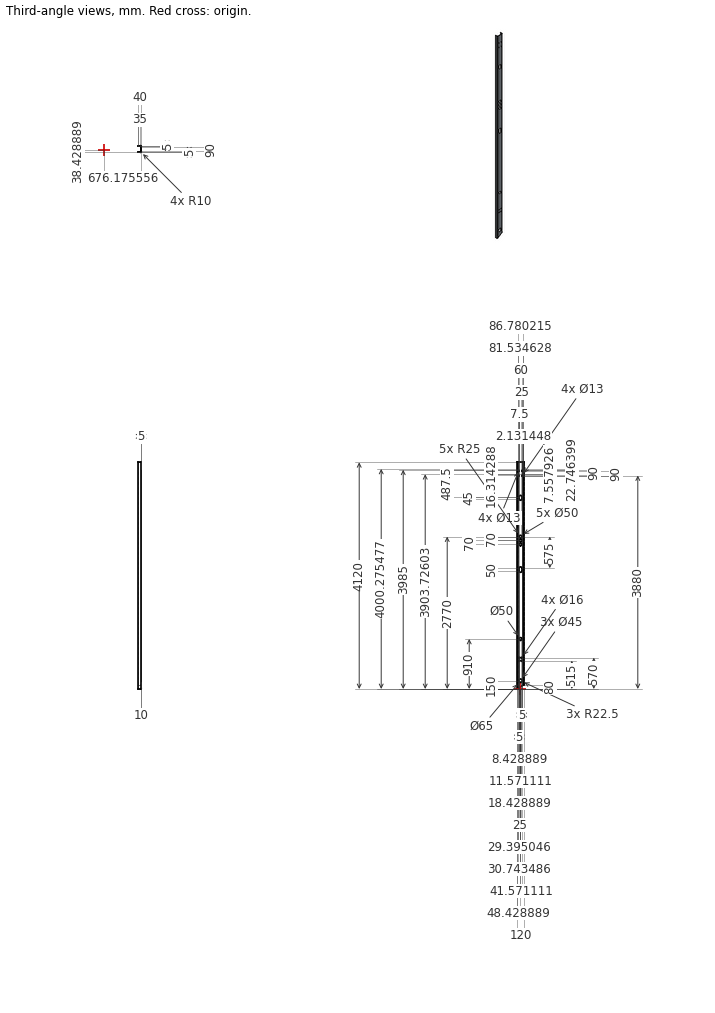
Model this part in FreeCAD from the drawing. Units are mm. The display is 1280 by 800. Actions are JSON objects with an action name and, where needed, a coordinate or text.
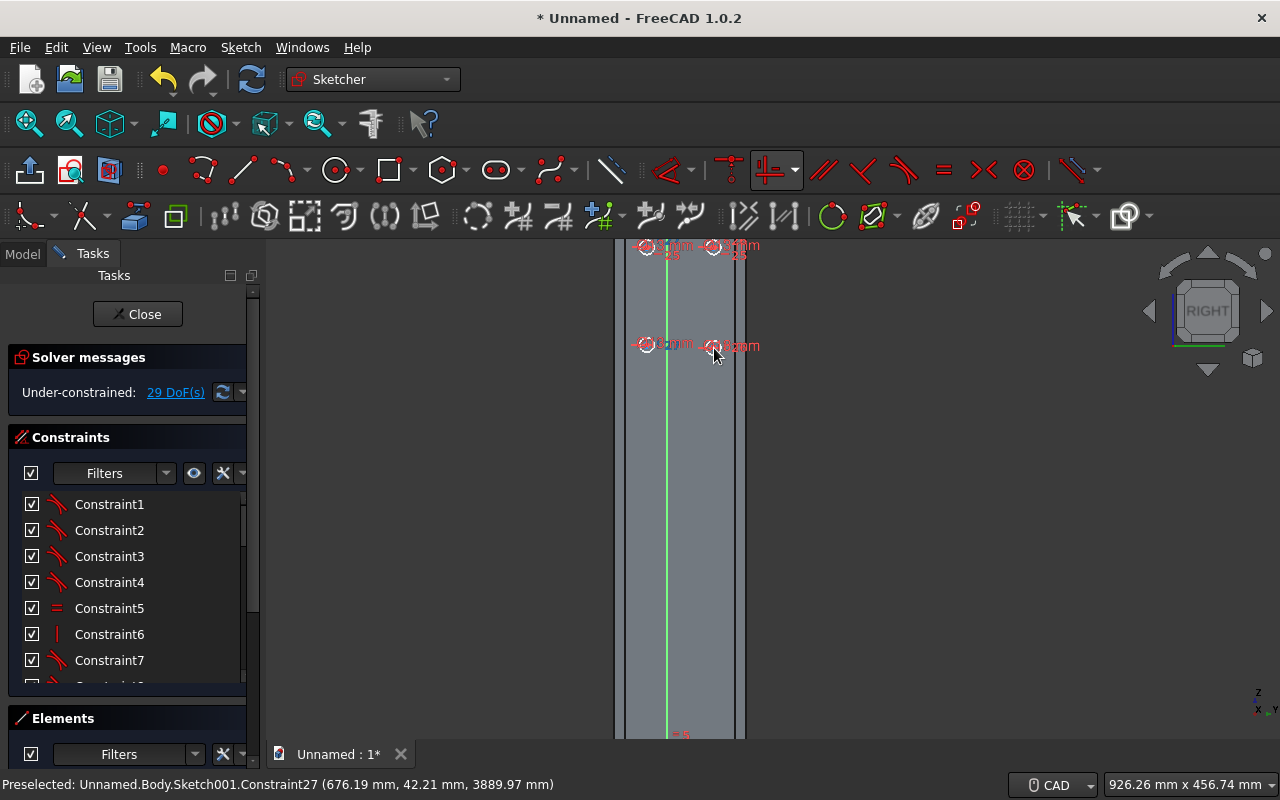
{"action": "left_click", "coordinate": [714, 348]}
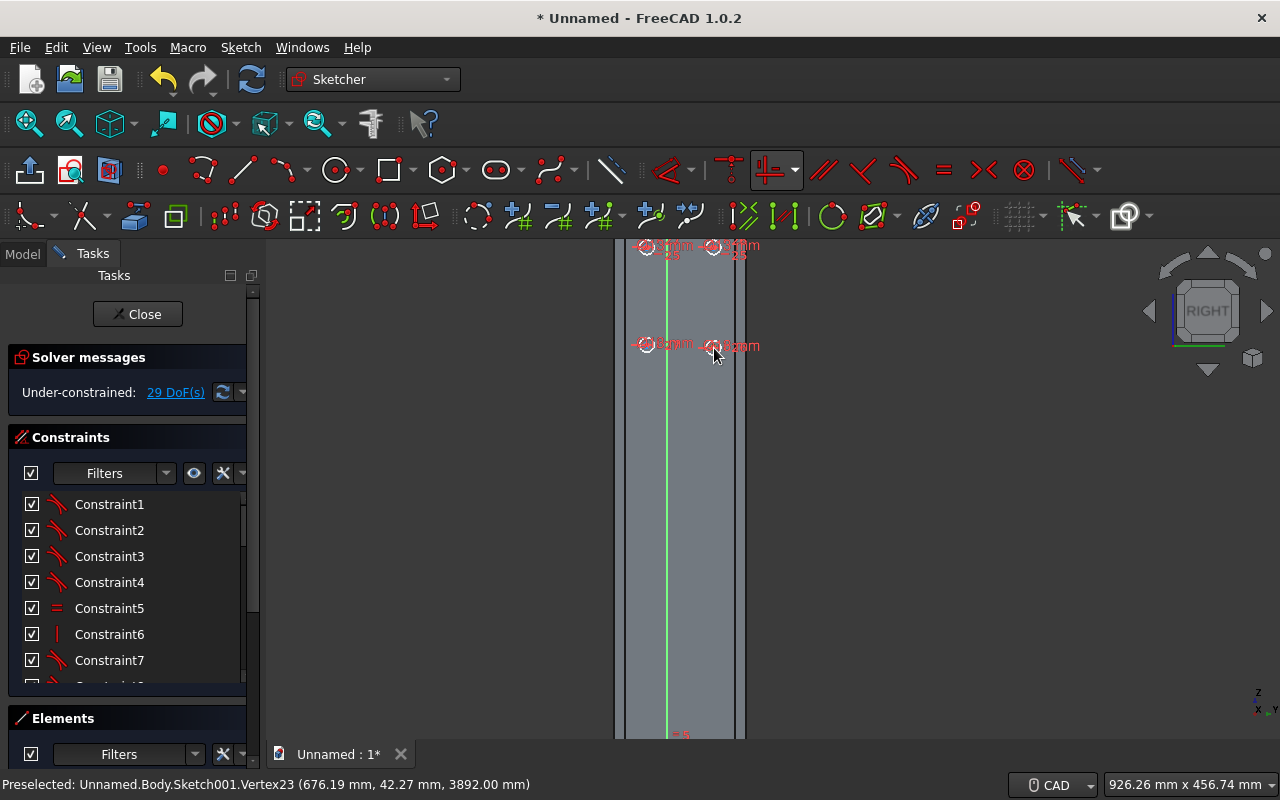
{"action": "scroll", "coordinate": [706, 334], "scroll_direction": "down", "scroll_amount": 13}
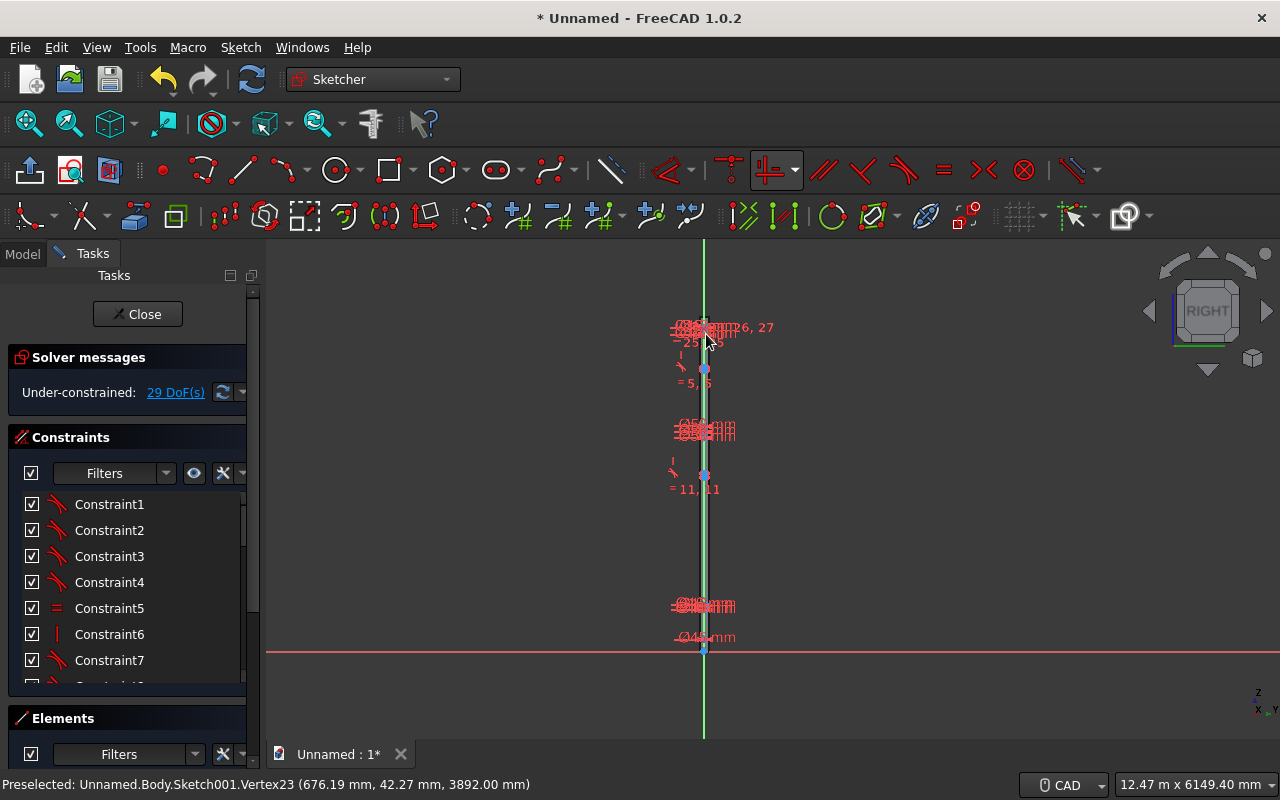
{"action": "scroll", "coordinate": [702, 335], "scroll_direction": "up", "scroll_amount": 5}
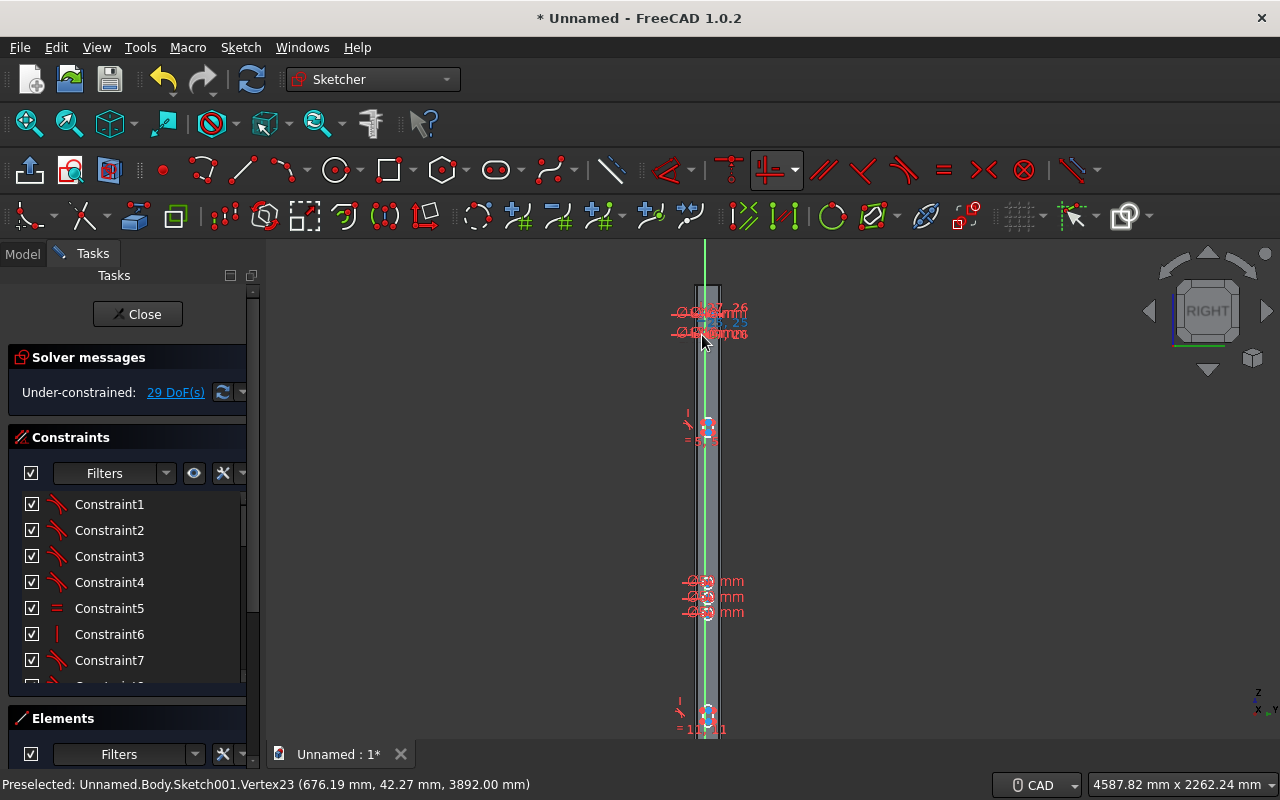
{"action": "scroll", "coordinate": [701, 335], "scroll_direction": "up", "scroll_amount": 4}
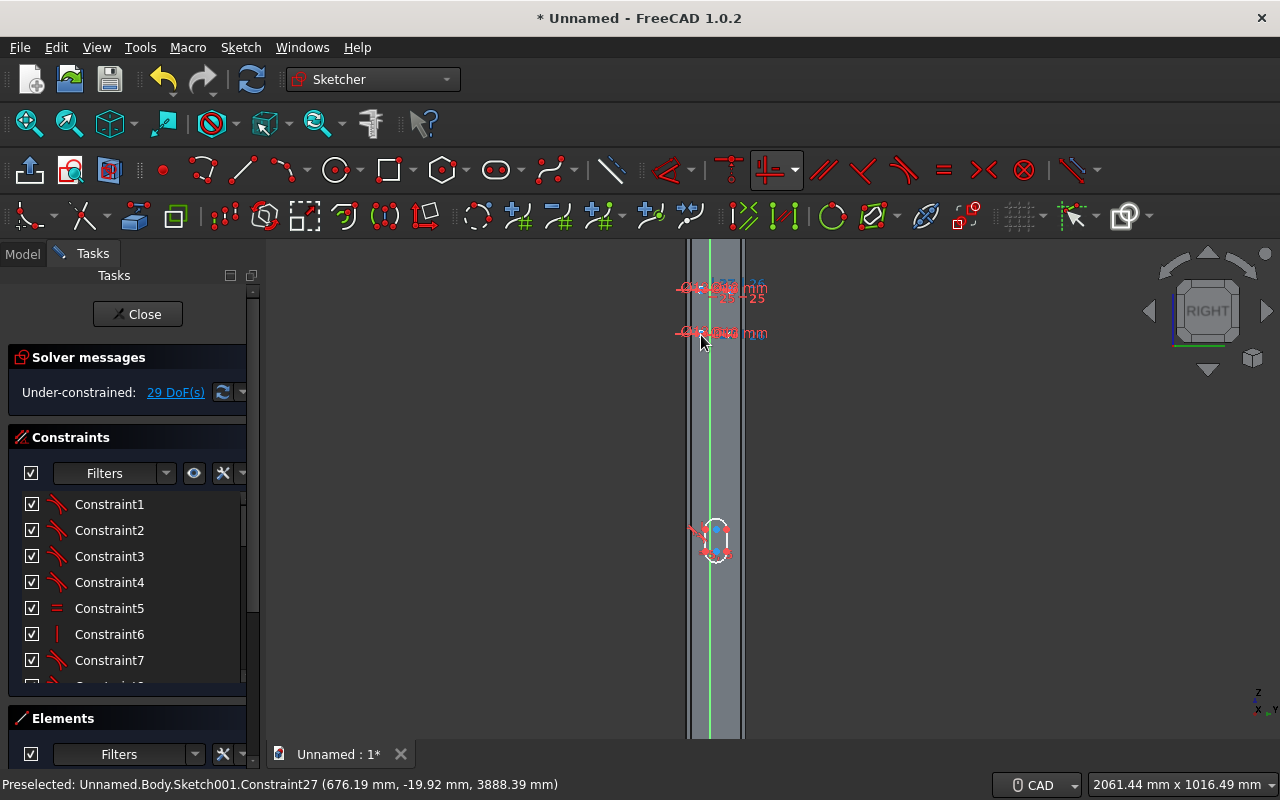
{"action": "left_click", "coordinate": [701, 334]}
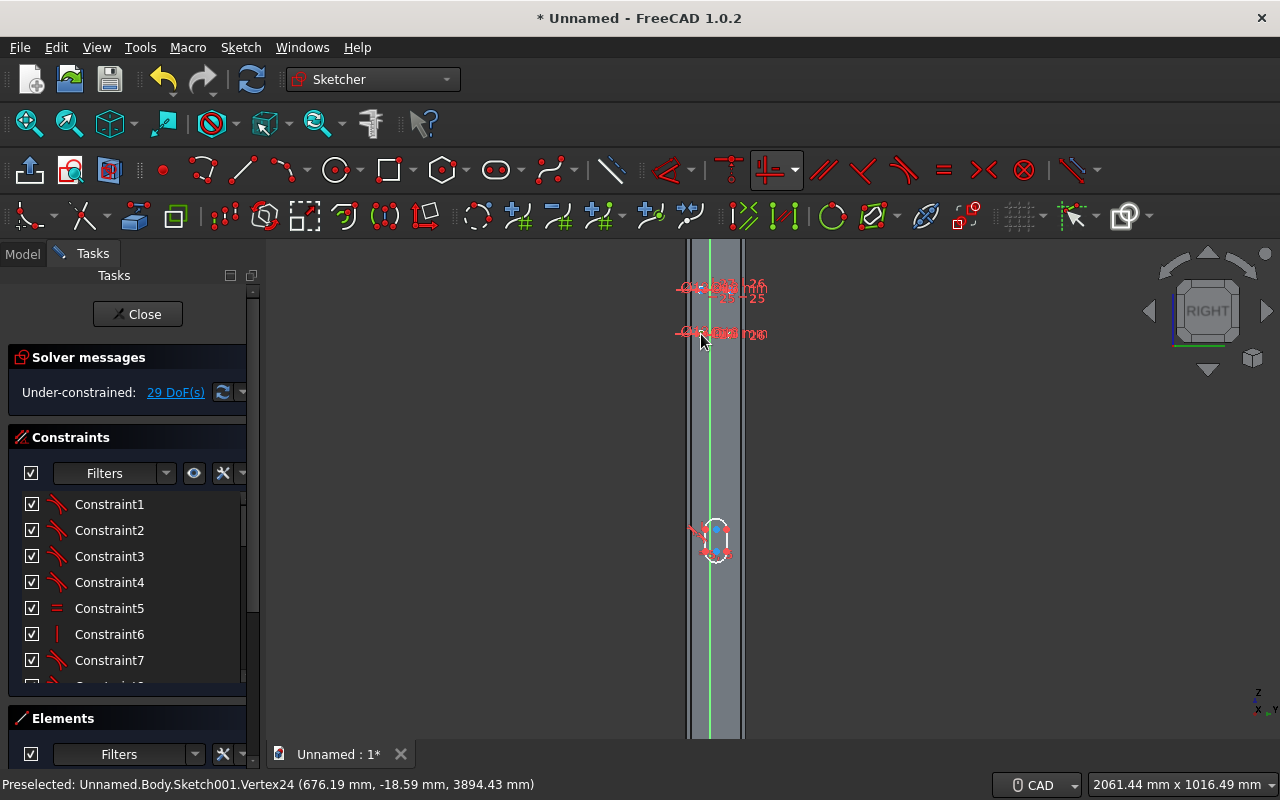
{"action": "left_click", "coordinate": [798, 170]}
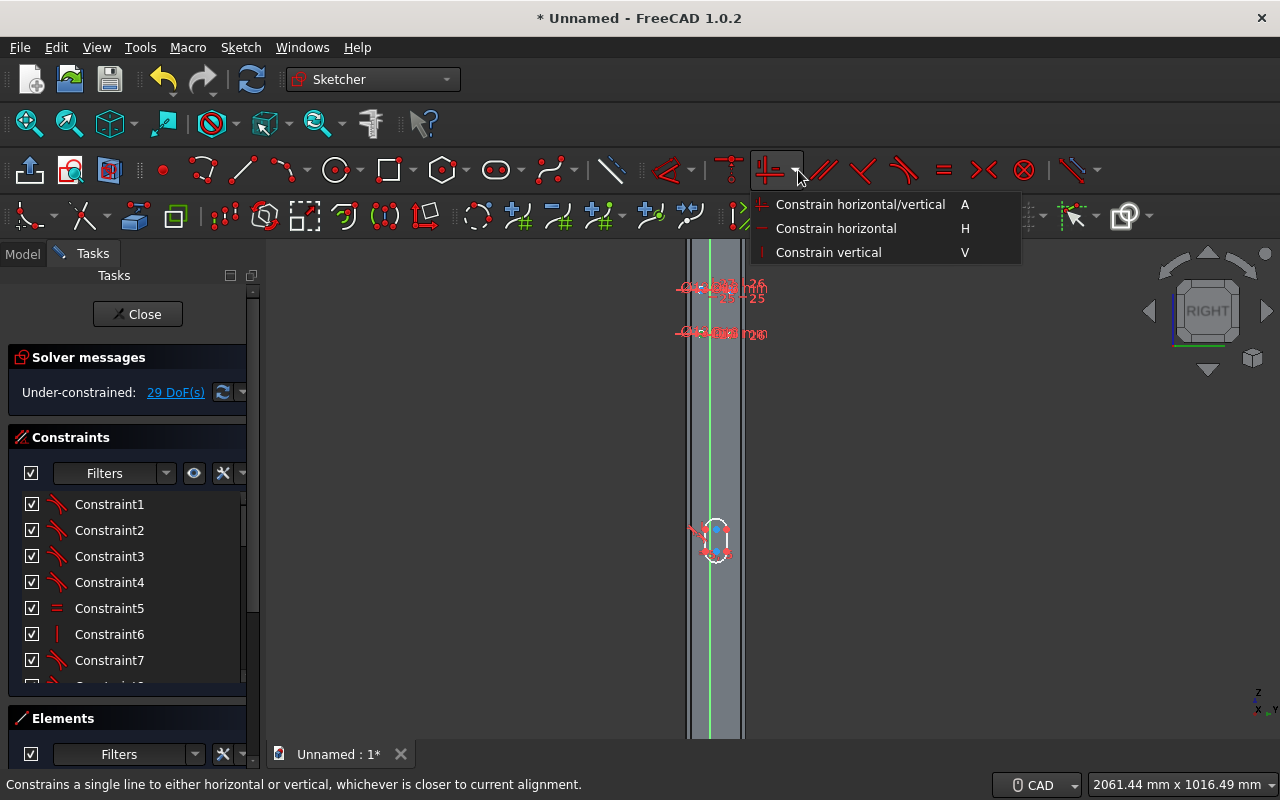
{"action": "left_click", "coordinate": [886, 228]}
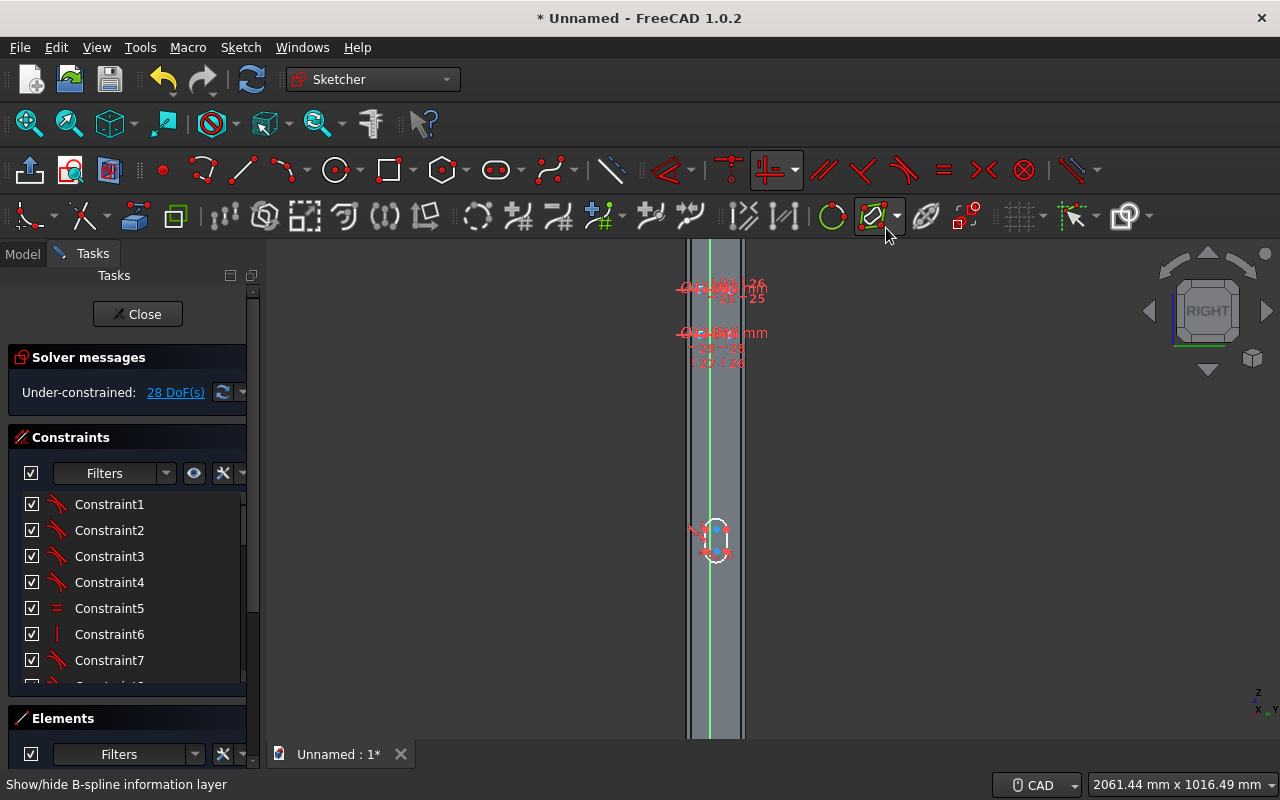
{"action": "scroll", "coordinate": [702, 335], "scroll_direction": "down", "scroll_amount": 9}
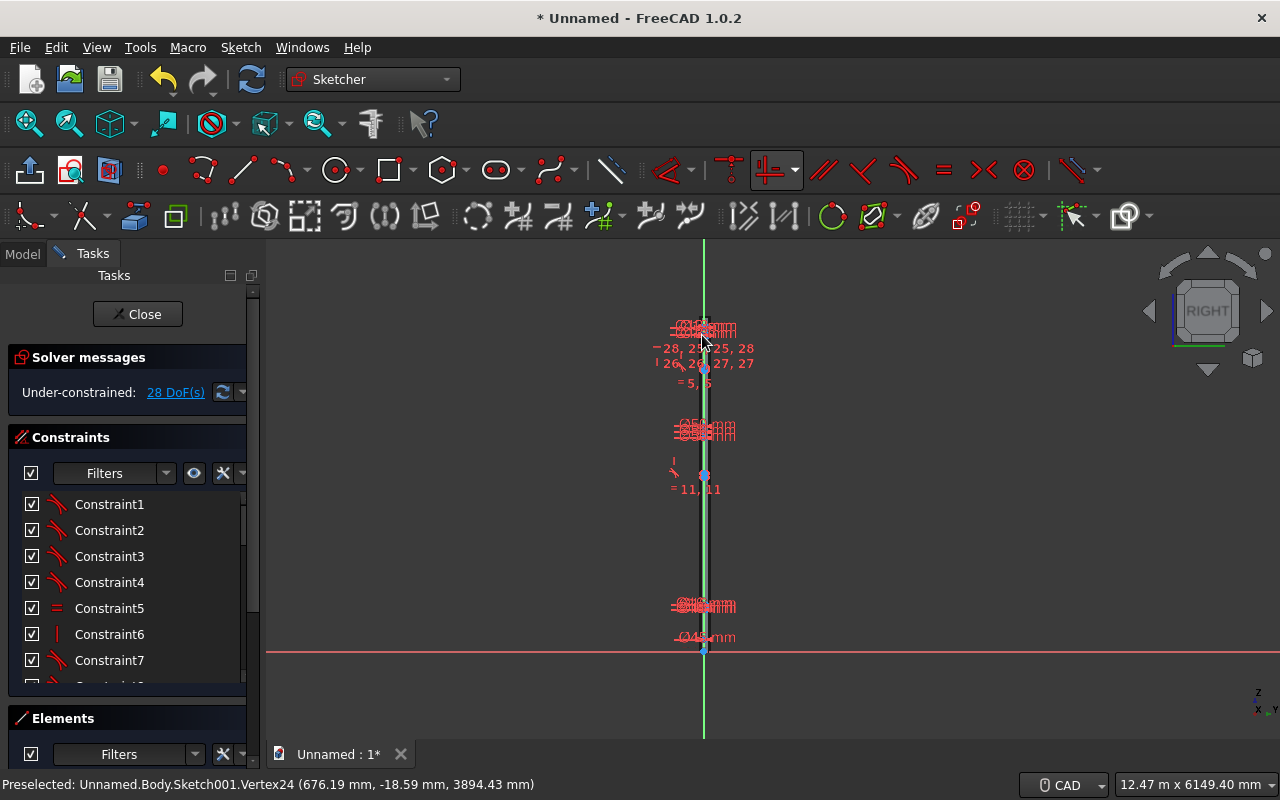
{"action": "scroll", "coordinate": [705, 426], "scroll_direction": "up", "scroll_amount": 4}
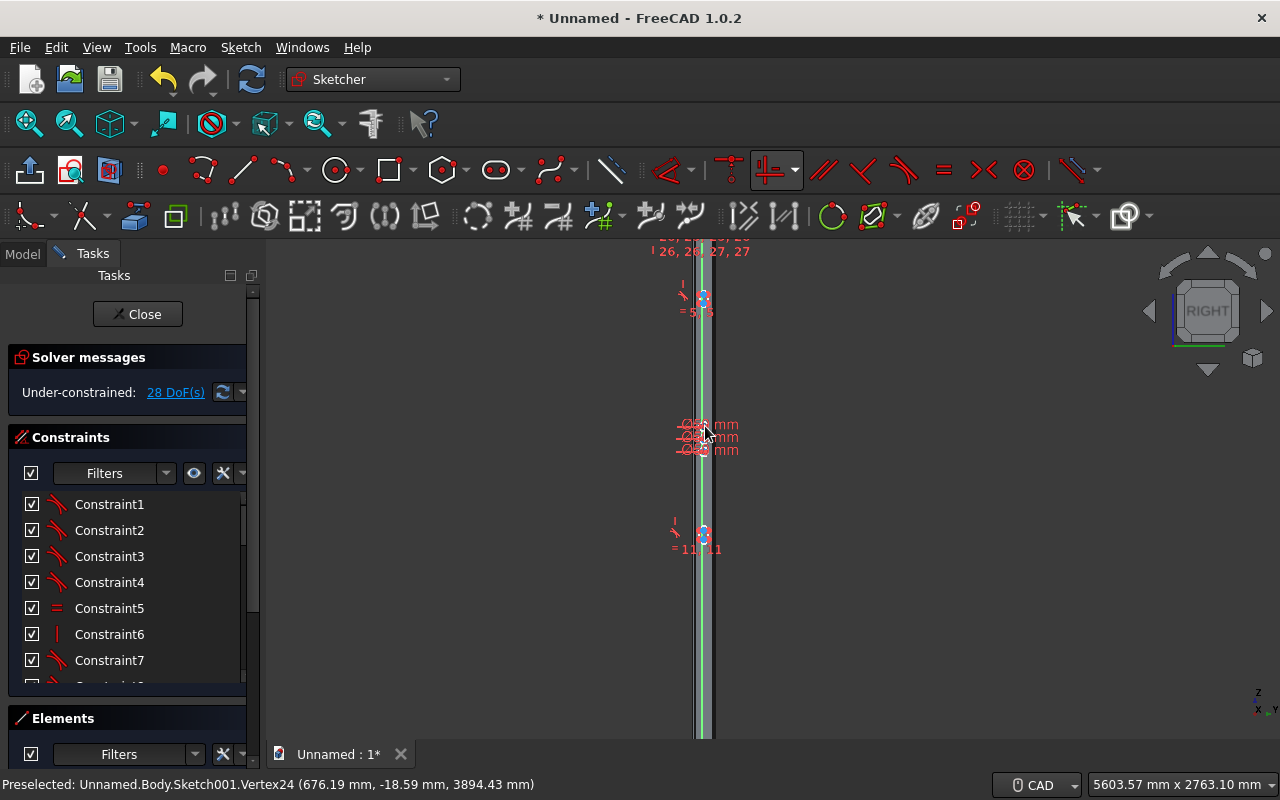
{"action": "left_click", "coordinate": [704, 427]}